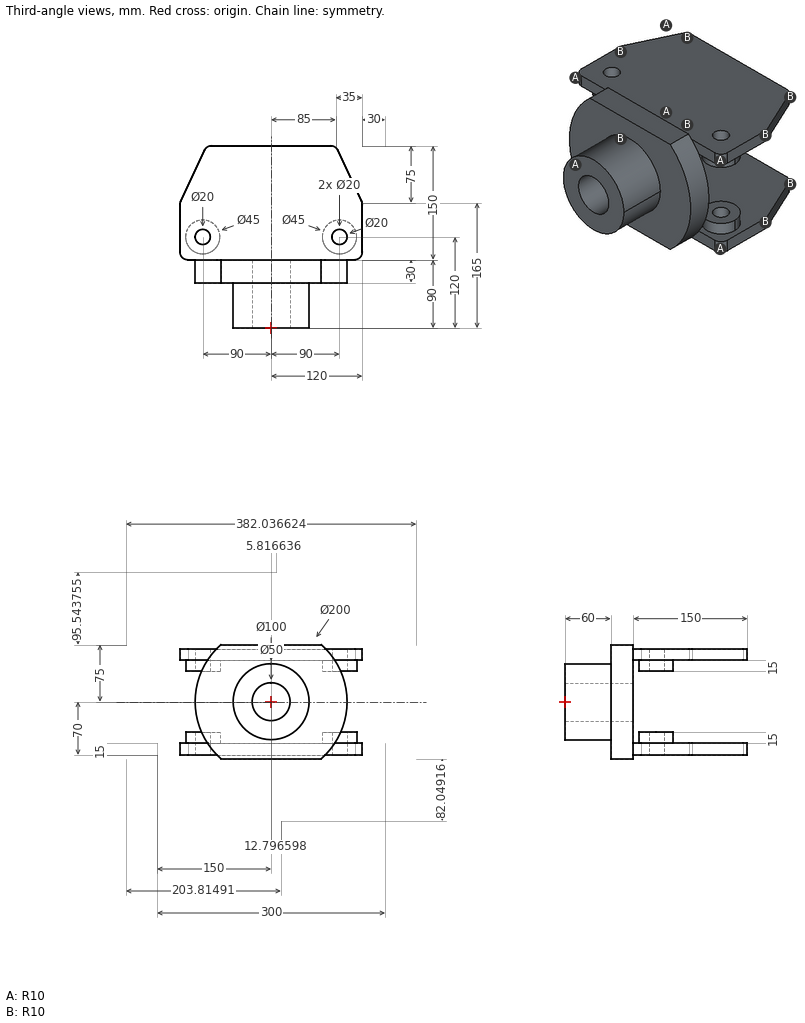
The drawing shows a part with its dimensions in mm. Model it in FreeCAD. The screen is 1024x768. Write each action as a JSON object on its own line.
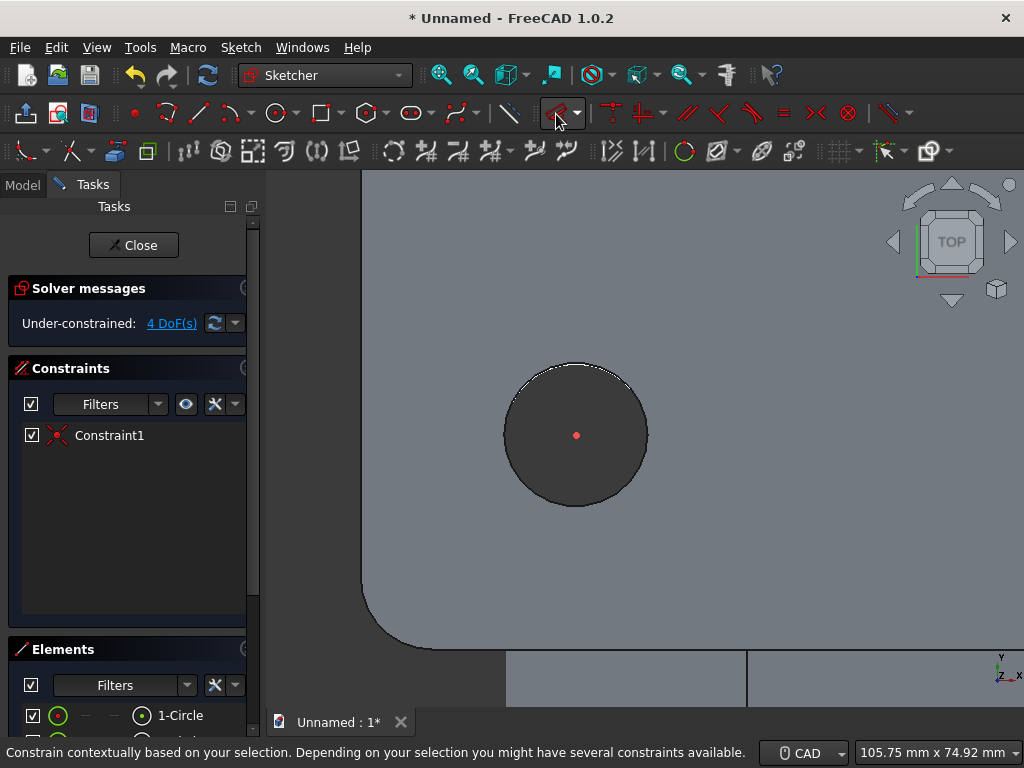
{"action": "left_click", "coordinate": [690, 322]}
{"action": "left_click", "coordinate": [713, 299]}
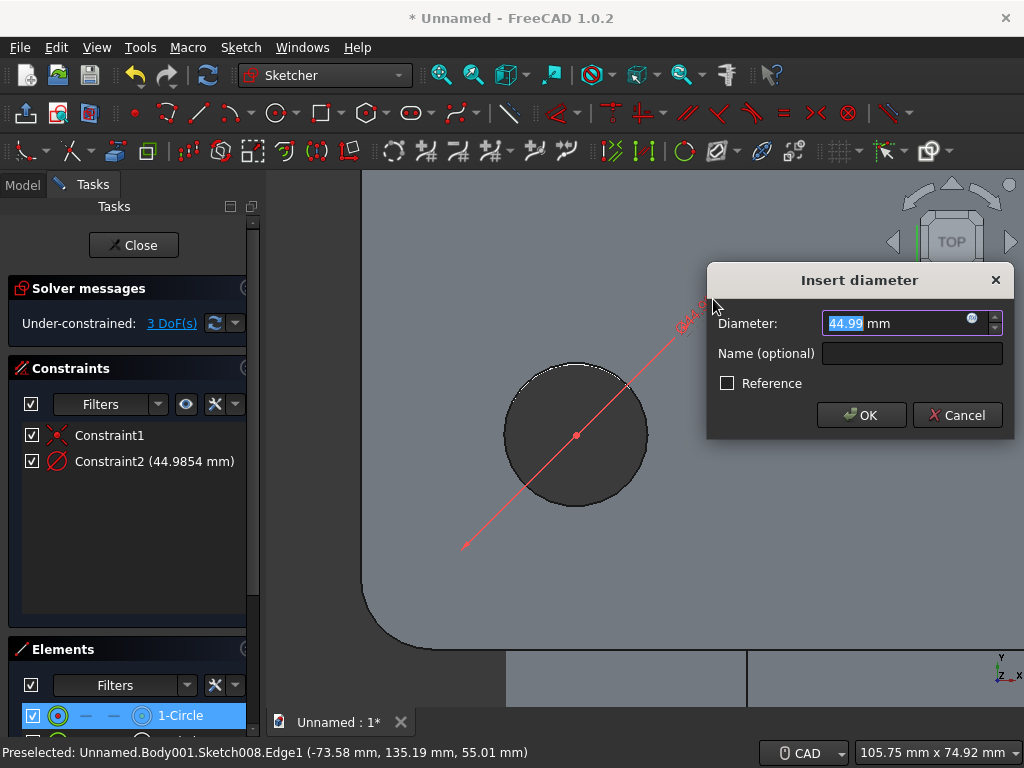
{"action": "type", "text": "45"}
{"action": "key", "text": "Return"}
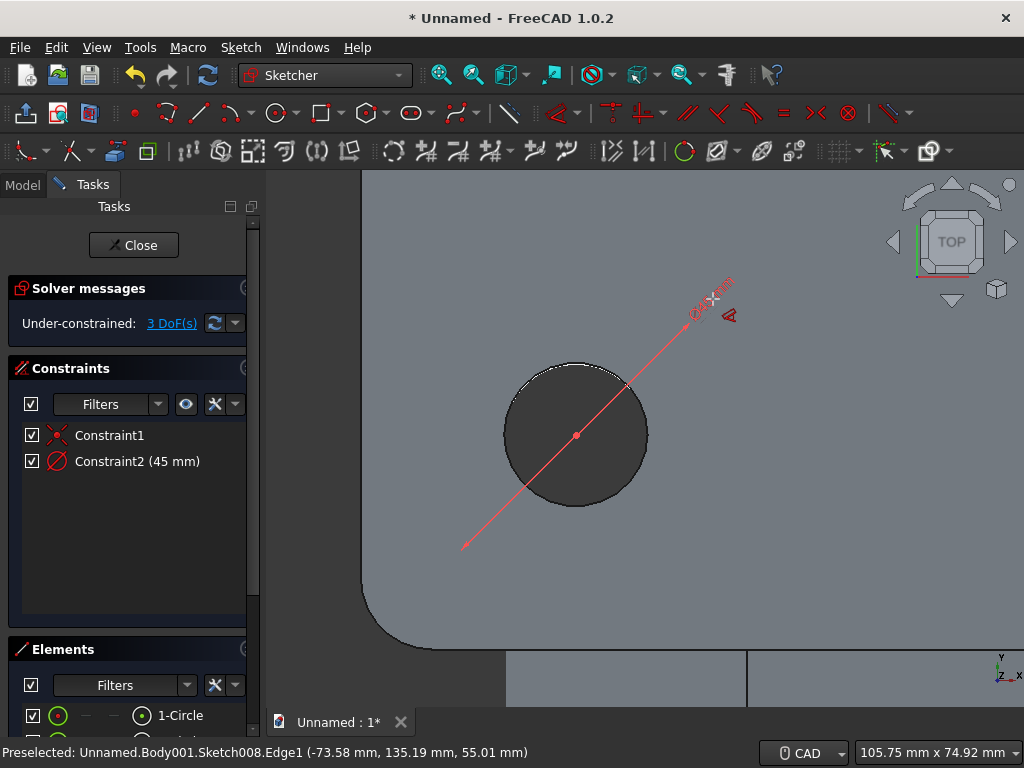
{"action": "left_click", "coordinate": [627, 385]}
{"action": "left_click", "coordinate": [650, 362]}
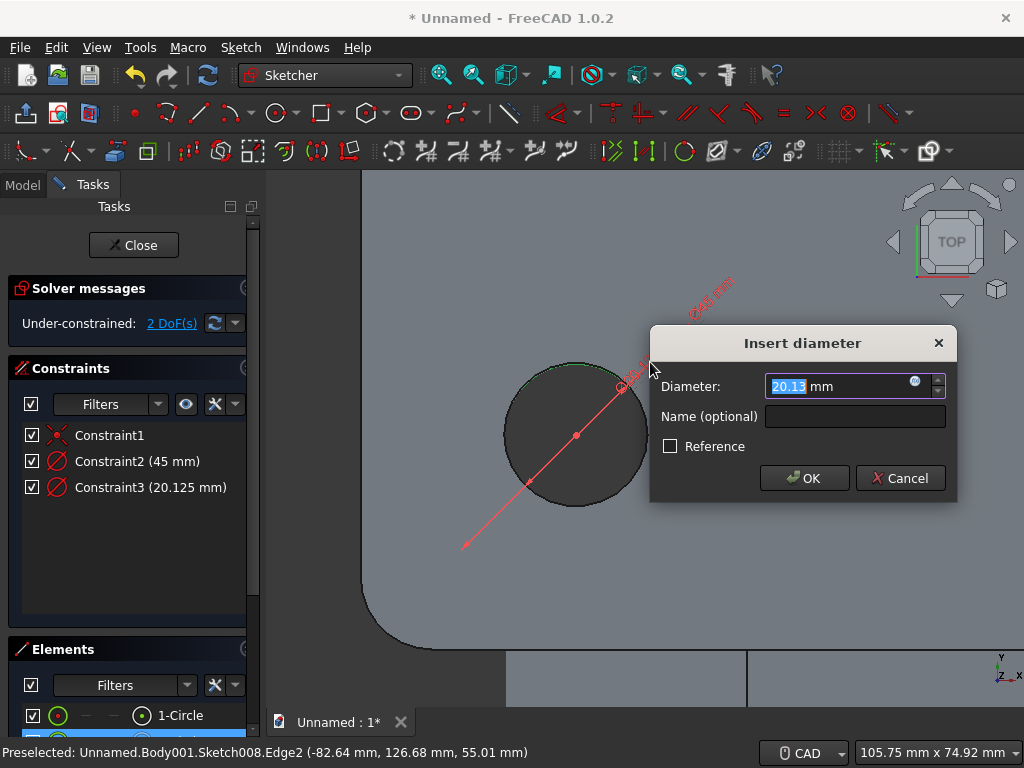
{"action": "type", "text": "20"}
{"action": "key", "text": "Return"}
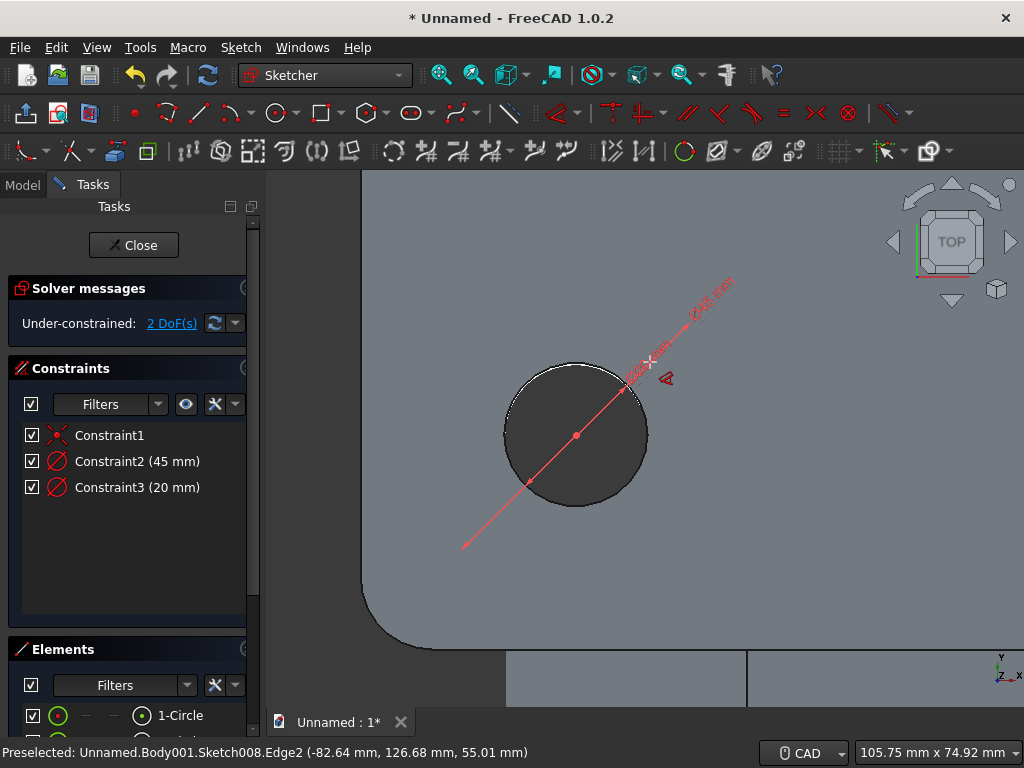
{"action": "left_click", "coordinate": [576, 436]}
{"action": "left_click", "coordinate": [718, 402]}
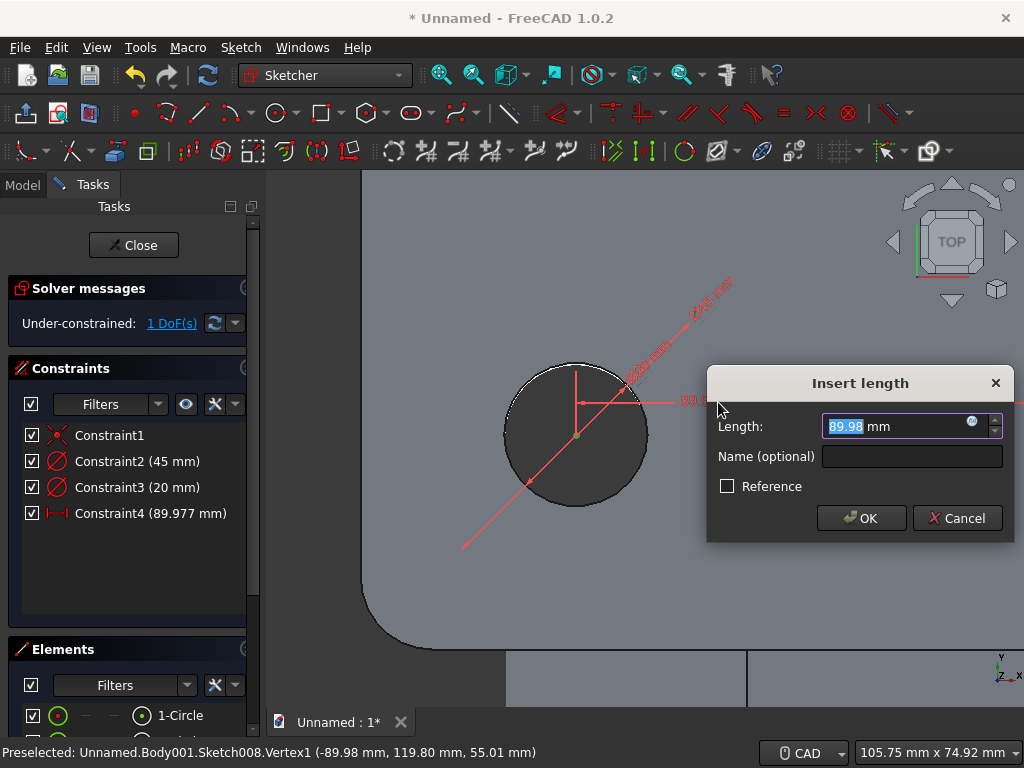
{"action": "type", "text": "90"}
{"action": "key", "text": "Return"}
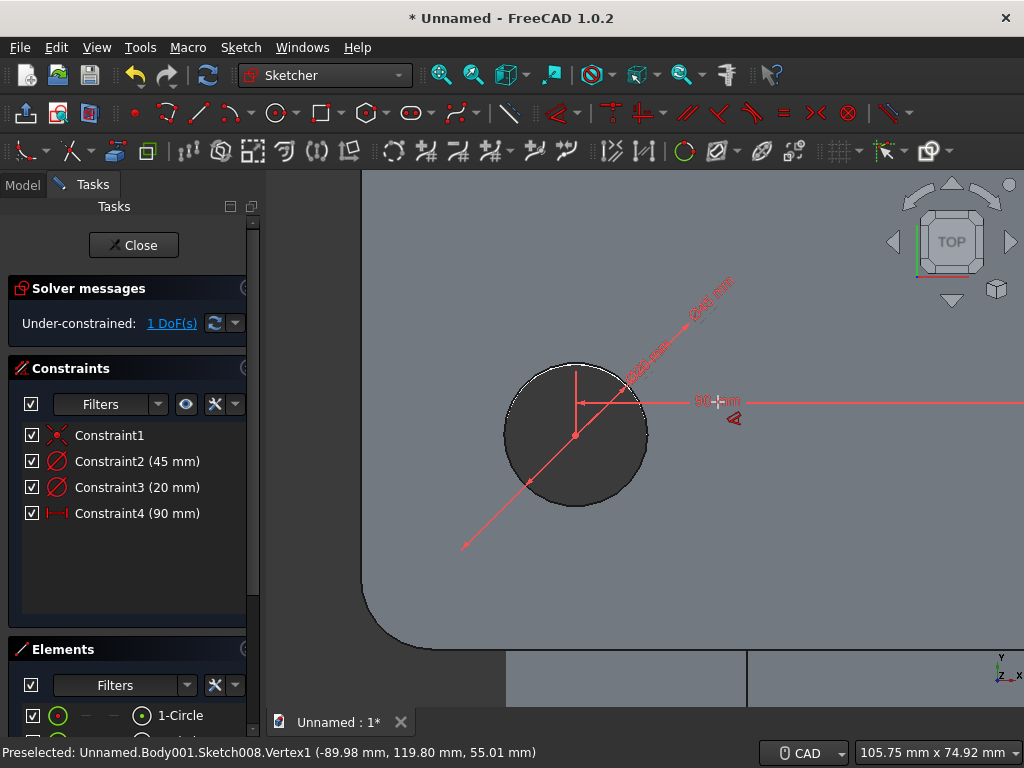
{"action": "left_click", "coordinate": [576, 436]}
{"action": "left_click", "coordinate": [542, 558]}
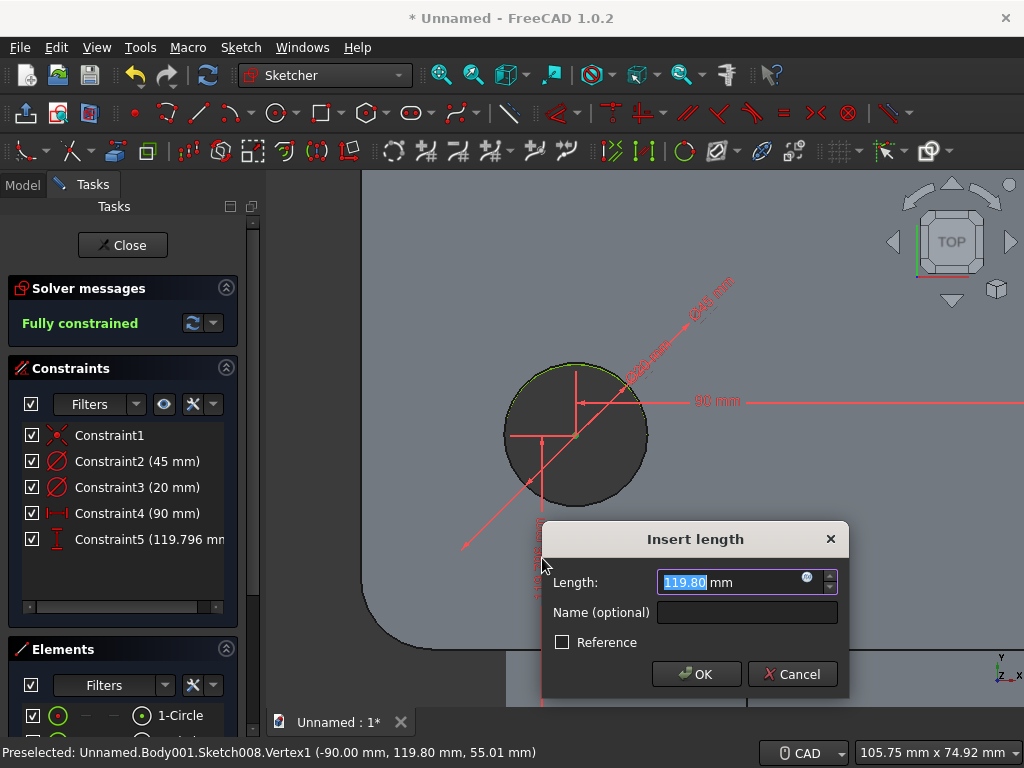
{"action": "type", "text": "120"}
{"action": "key", "text": "Return"}
{"action": "key", "text": "Escape"}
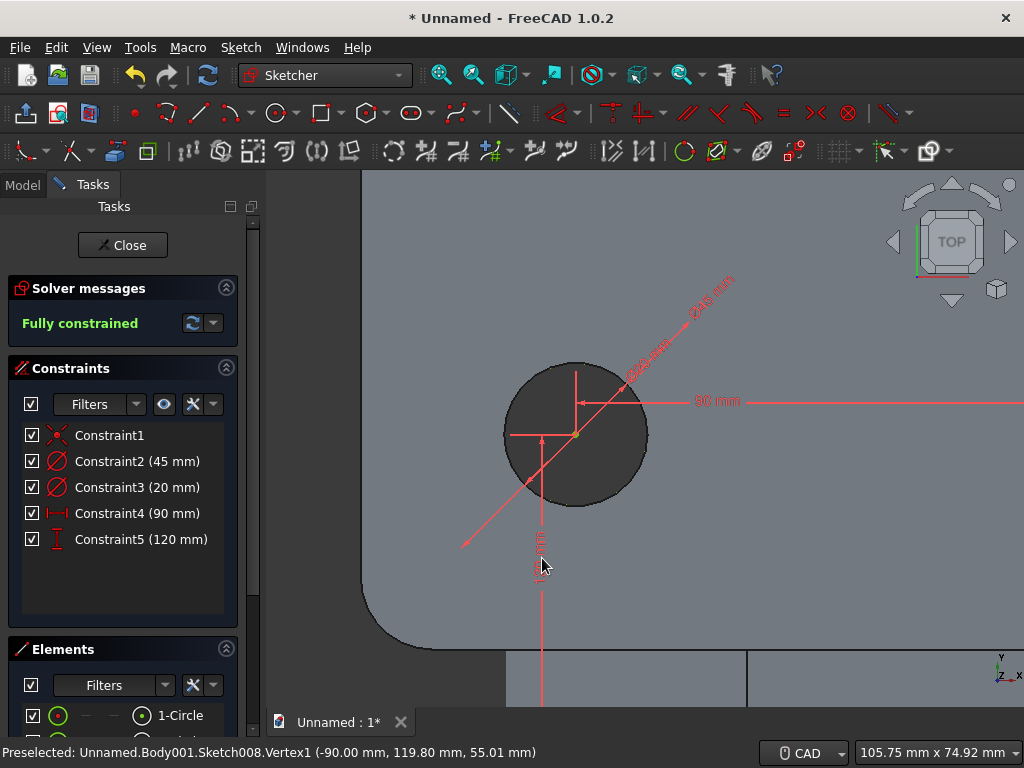
{"action": "left_click", "coordinate": [123, 245]}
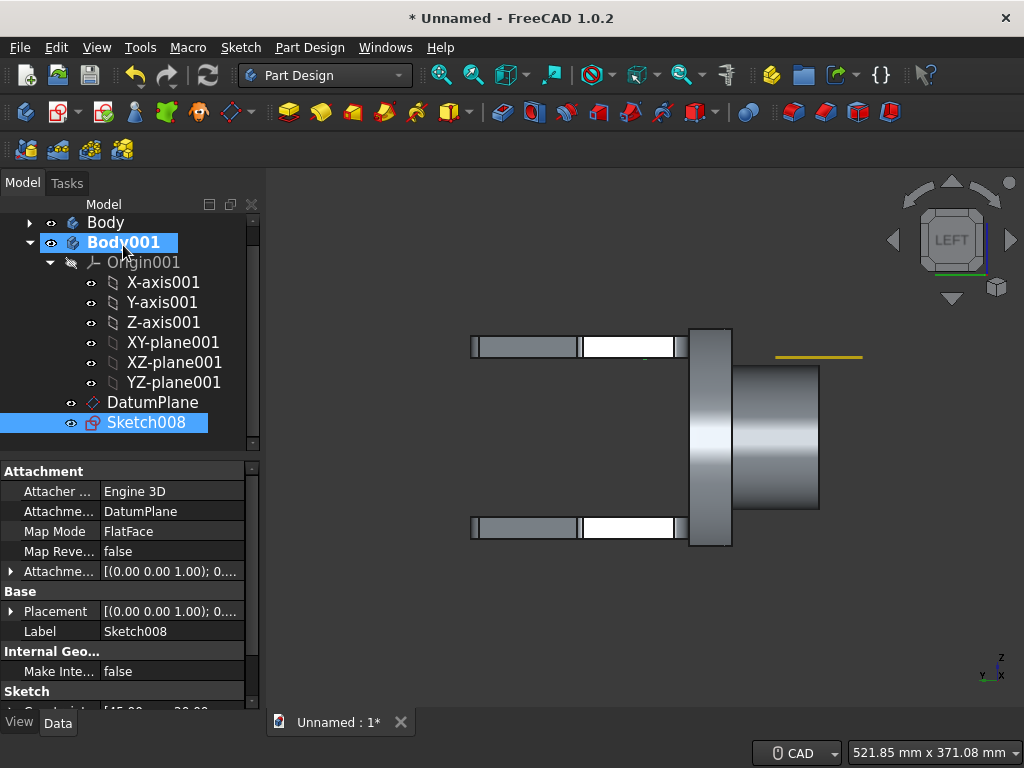
{"action": "left_click", "coordinate": [290, 112]}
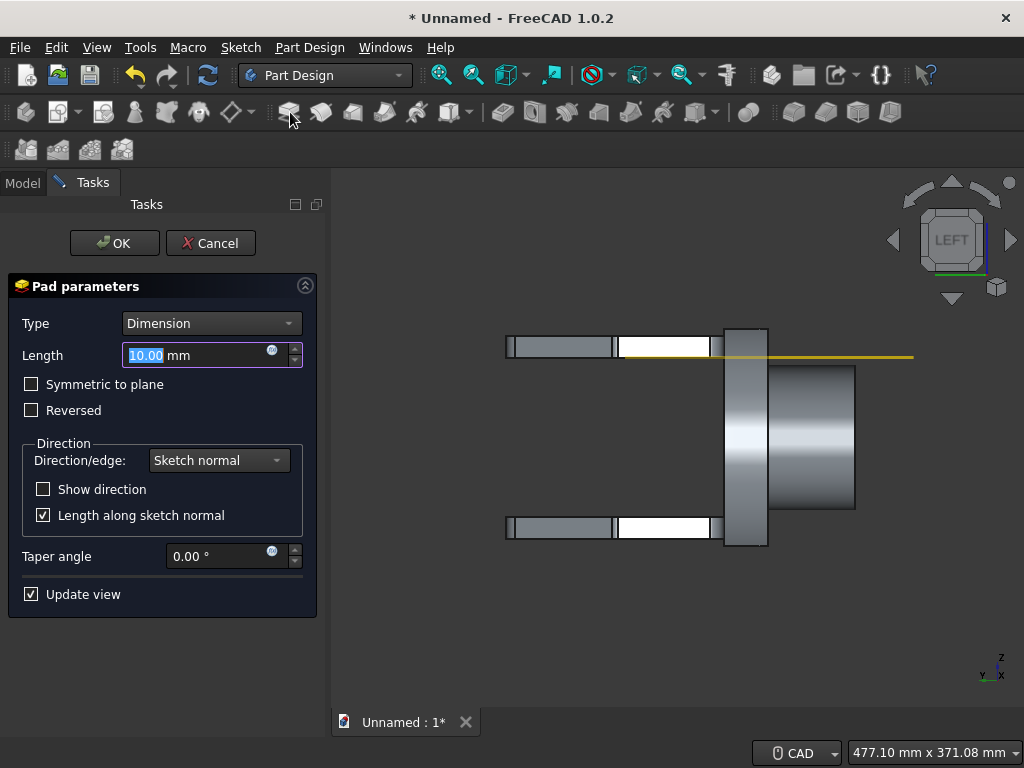
{"action": "type", "text": "15"}
{"action": "key", "text": "Tab"}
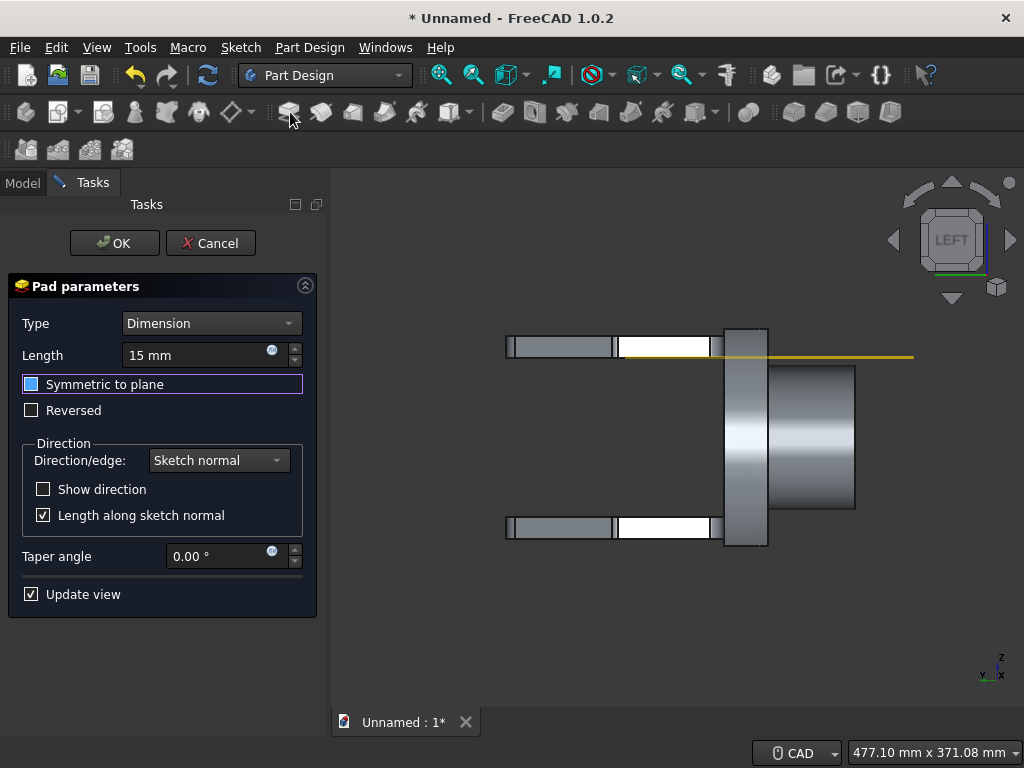
{"action": "left_click", "coordinate": [30, 410]}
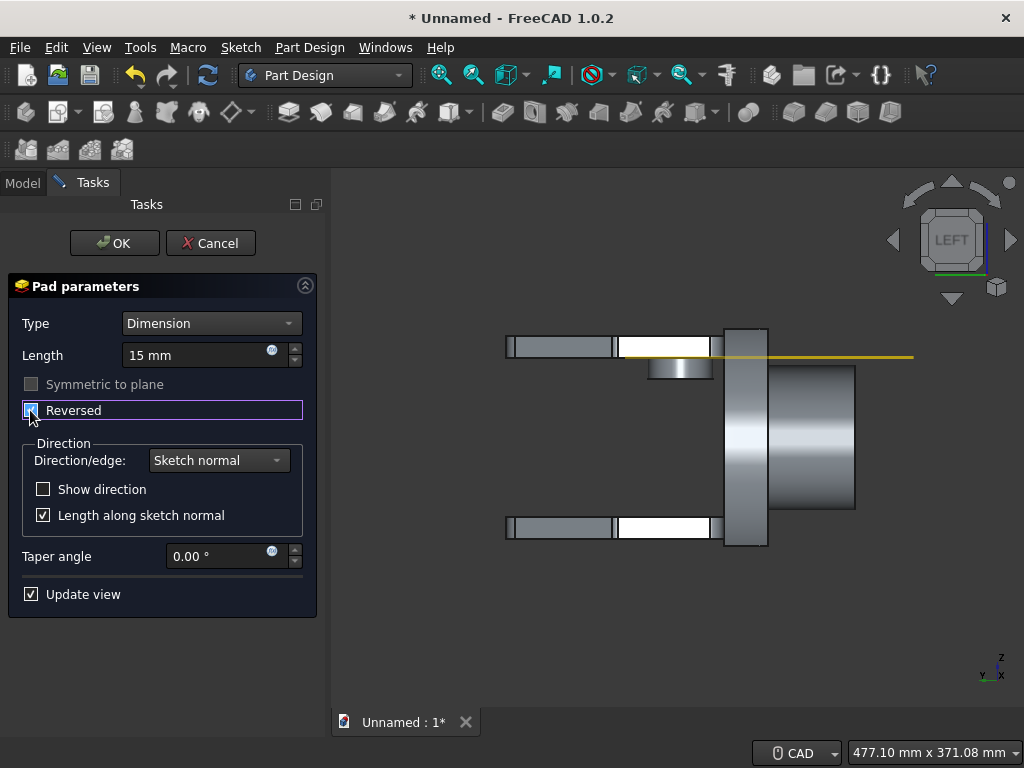
{"action": "left_click", "coordinate": [115, 243]}